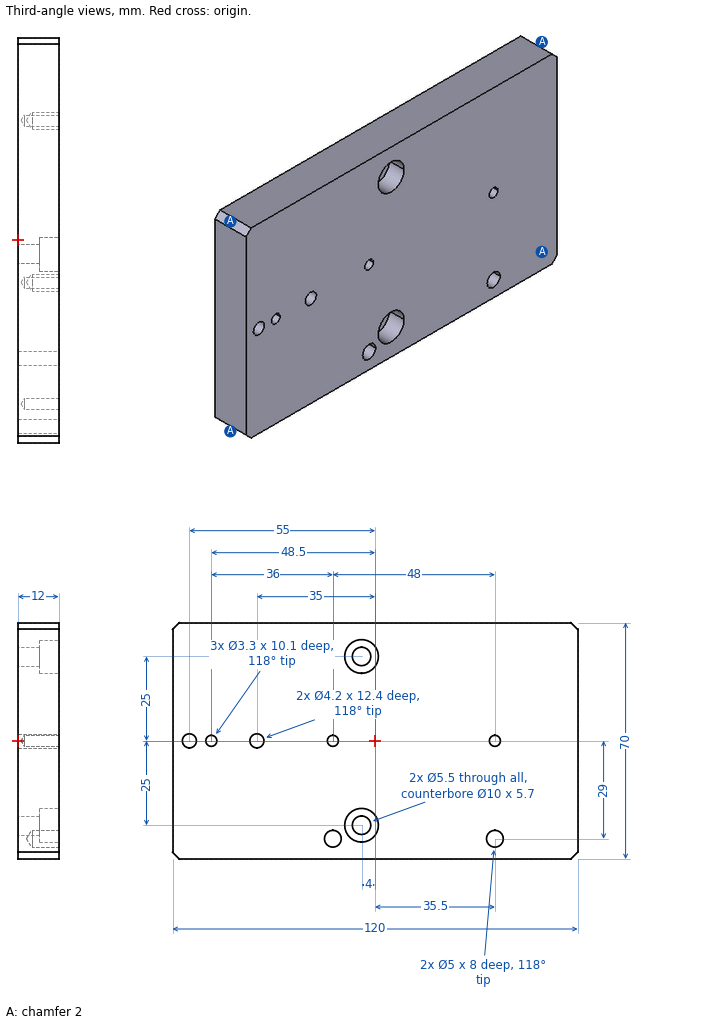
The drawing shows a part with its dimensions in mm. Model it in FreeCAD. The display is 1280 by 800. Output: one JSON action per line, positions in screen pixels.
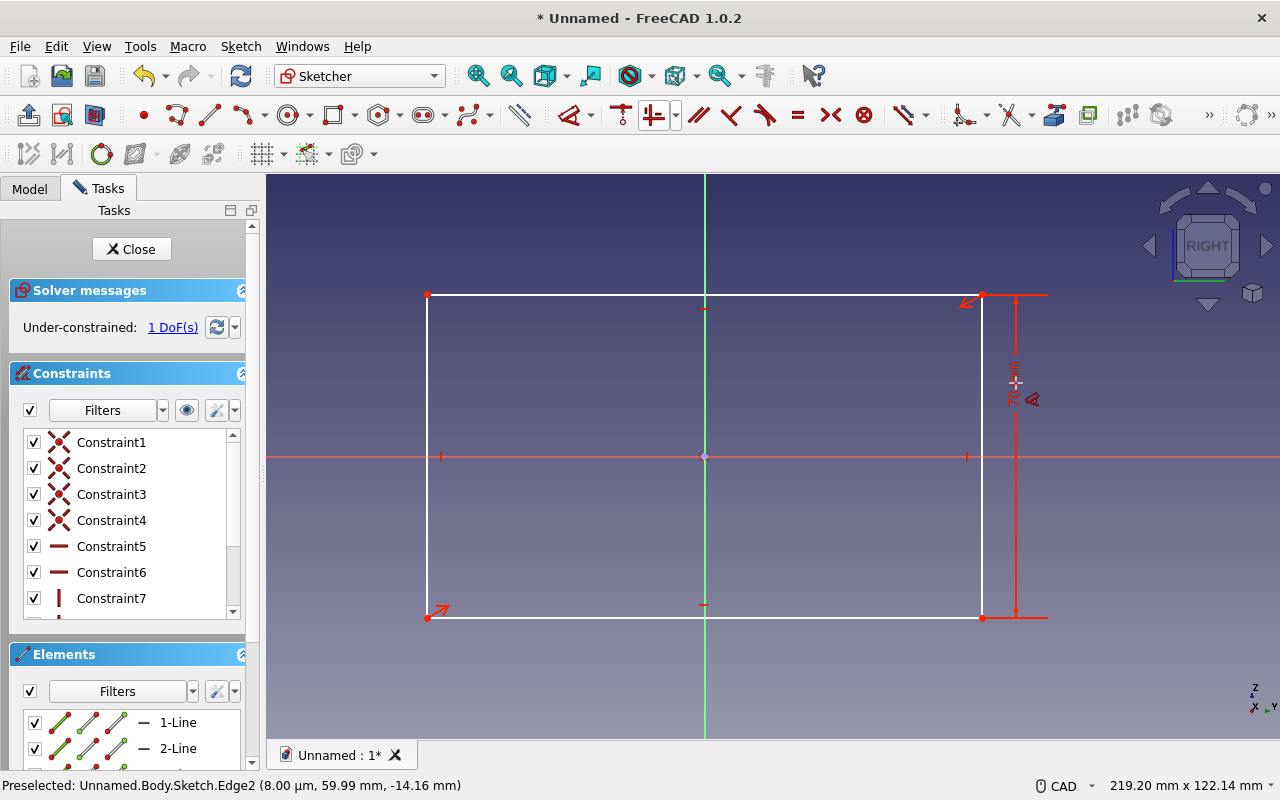
{"action": "left_click", "coordinate": [594, 618]}
{"action": "left_click", "coordinate": [577, 652]}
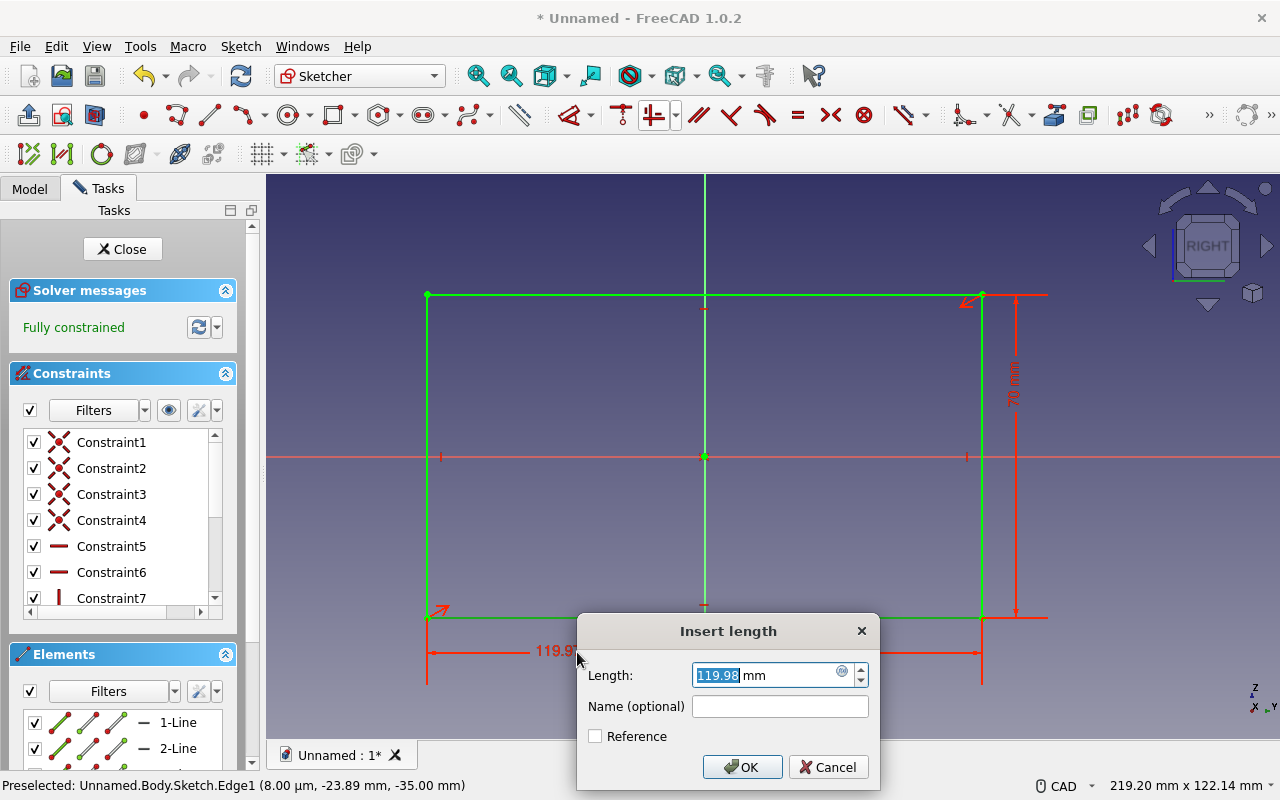
{"action": "type", "text": "120"}
{"action": "key", "text": "Return"}
{"action": "key", "text": "Escape"}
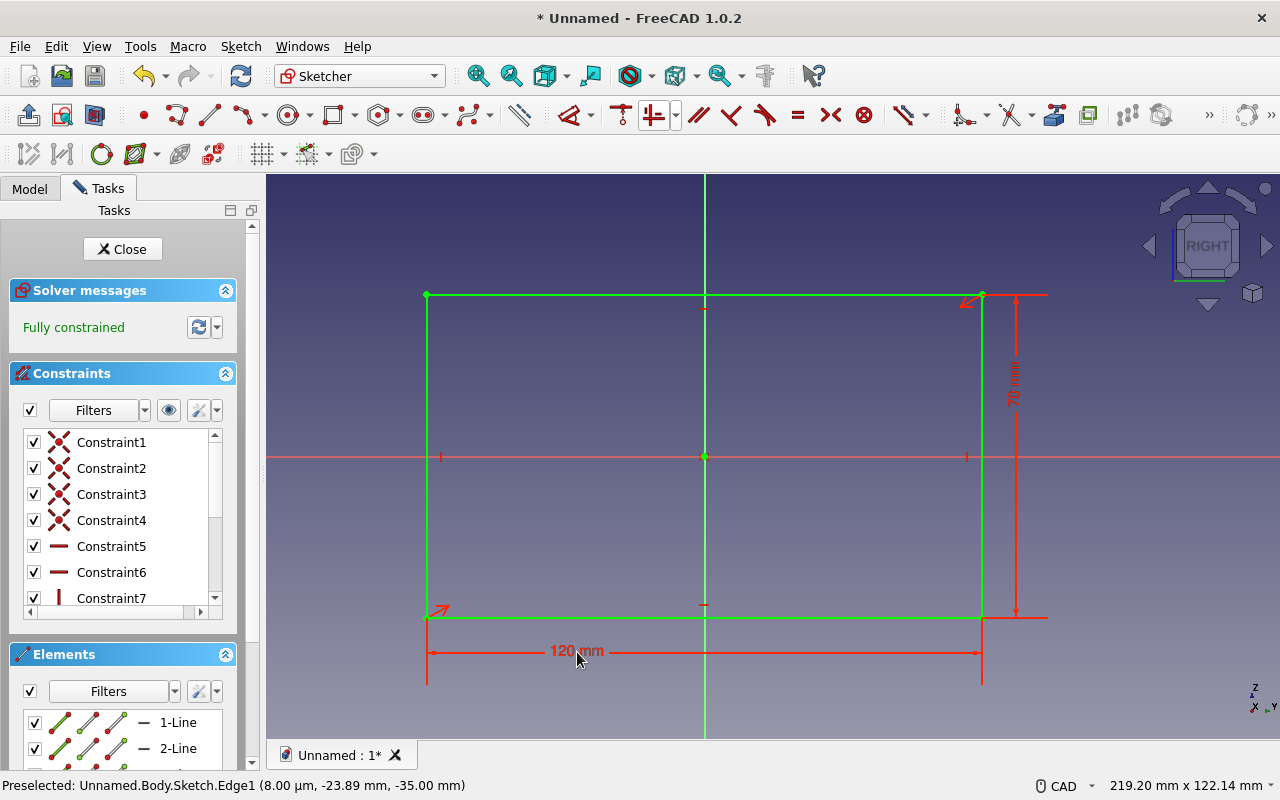
{"action": "left_click", "coordinate": [123, 249]}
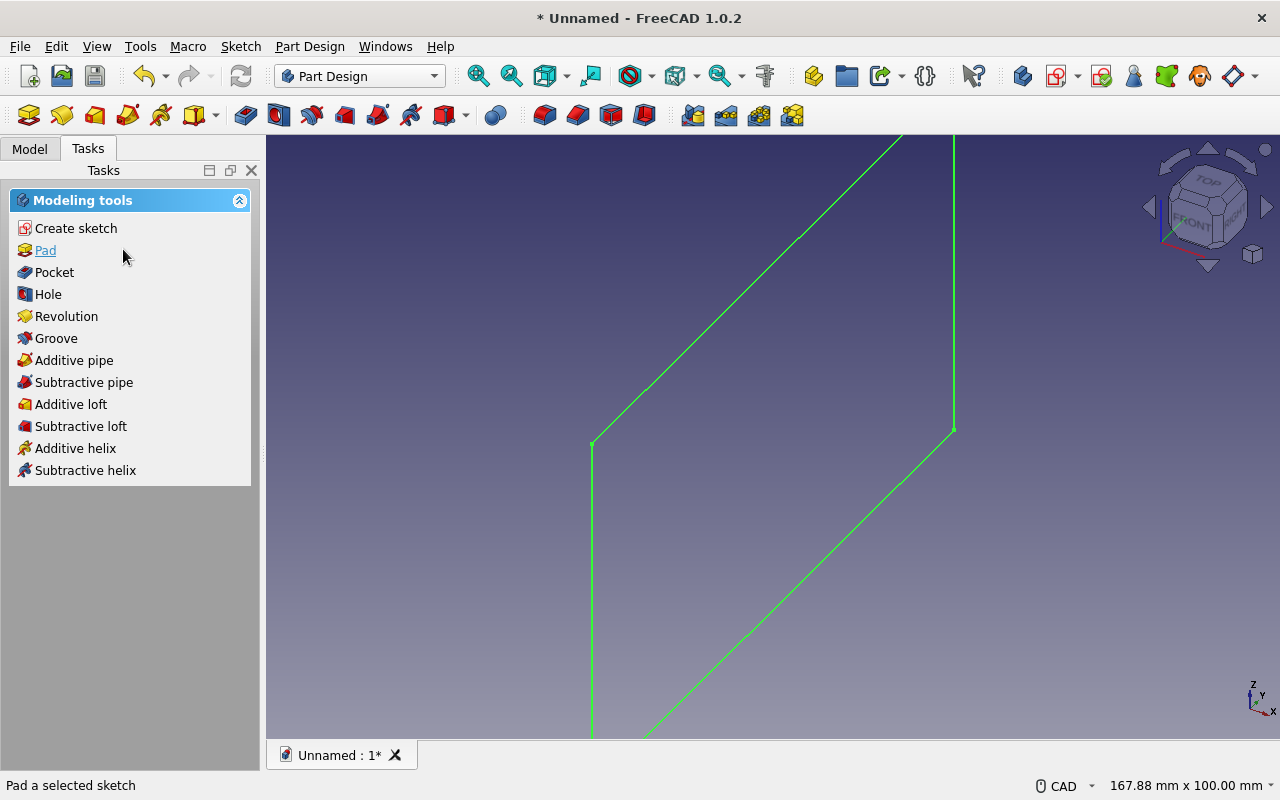
{"action": "left_click", "coordinate": [29, 116]}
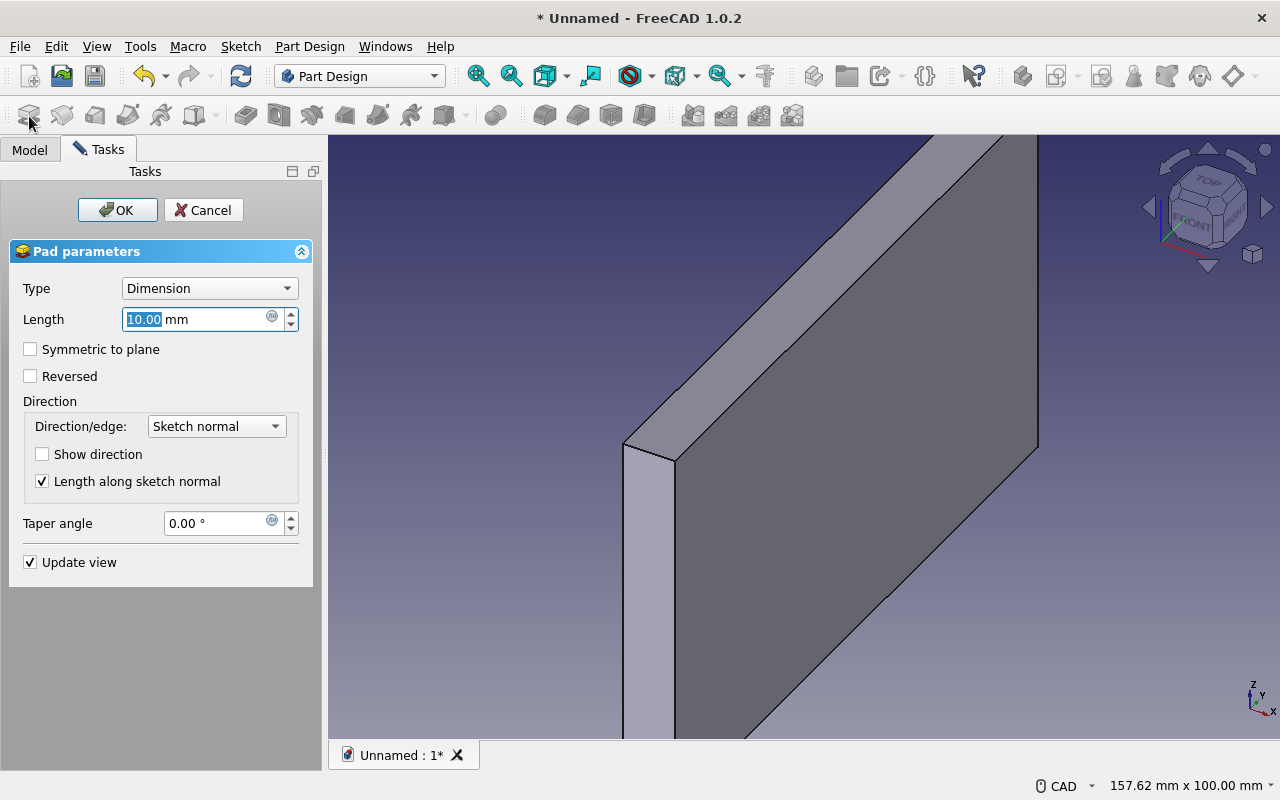
{"action": "type", "text": "12"}
{"action": "key", "text": "Tab"}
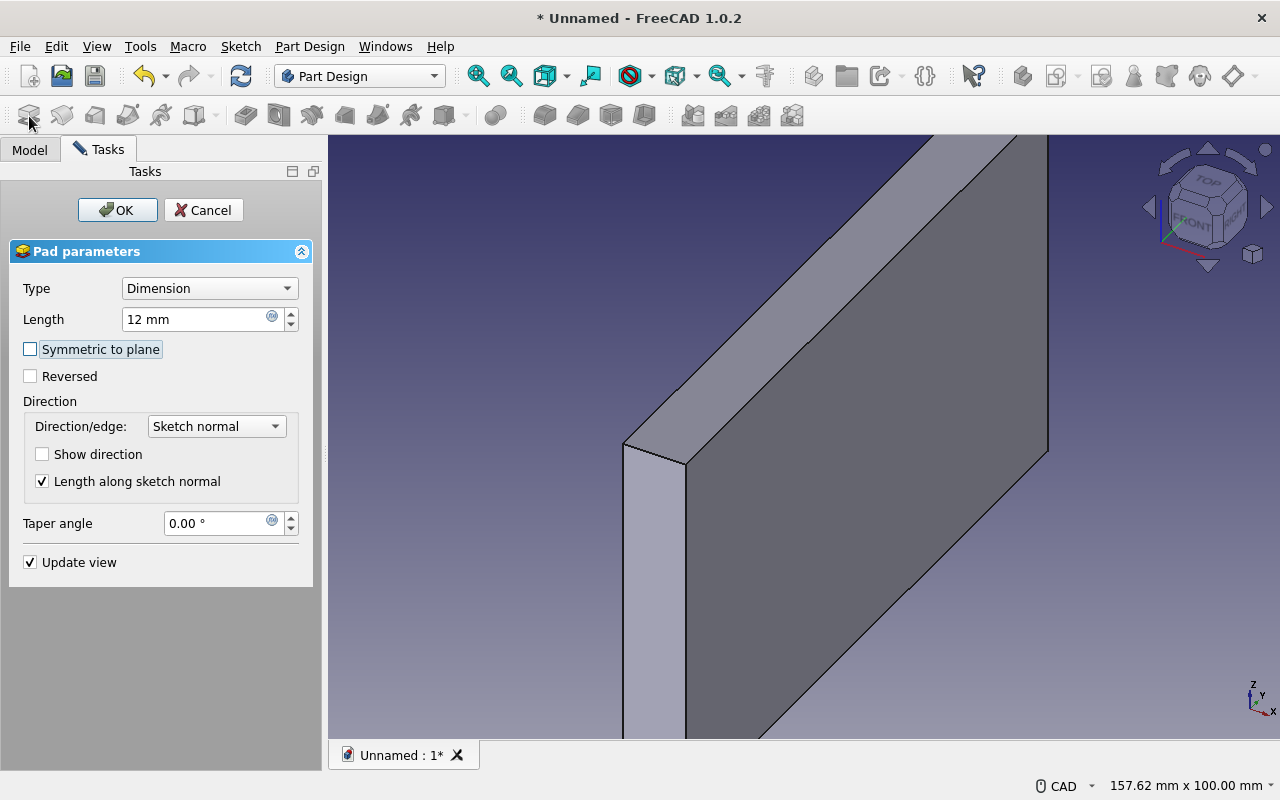
{"action": "left_click", "coordinate": [118, 210]}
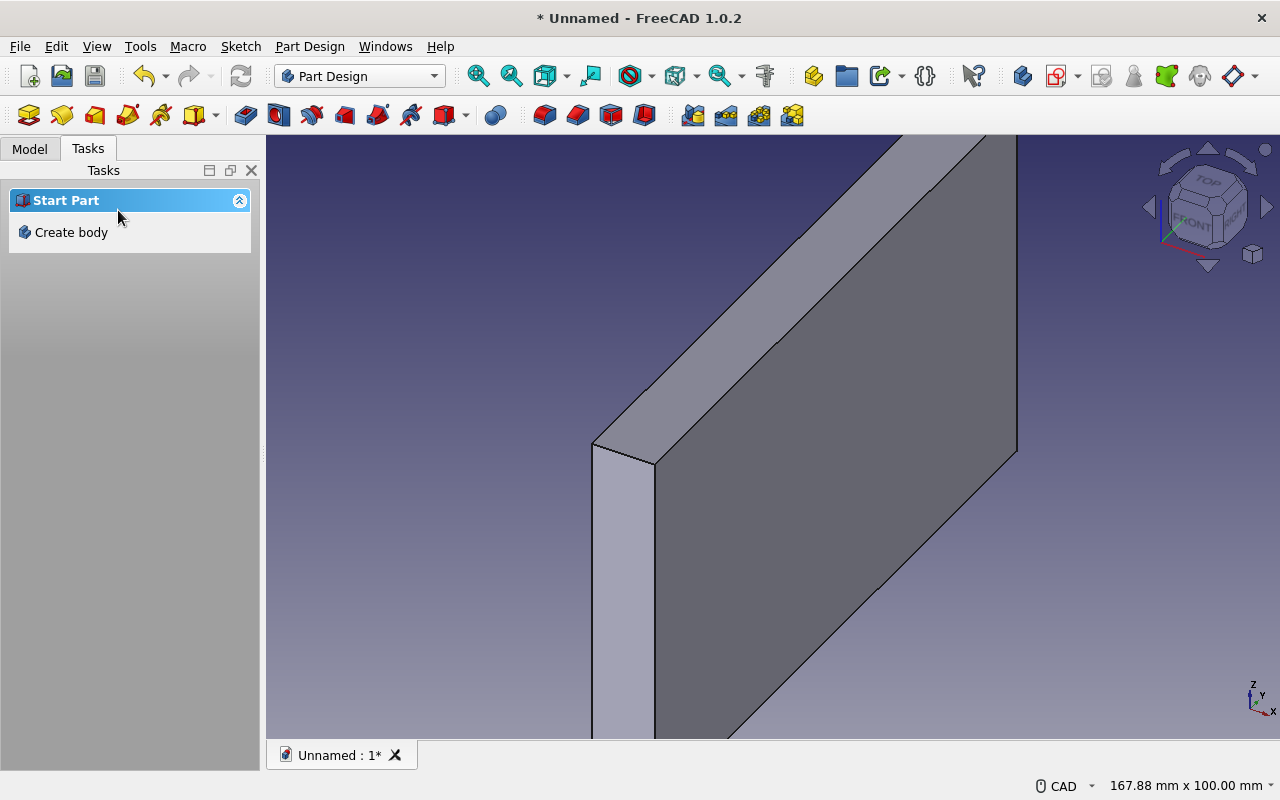
{"action": "left_click", "coordinate": [479, 76]}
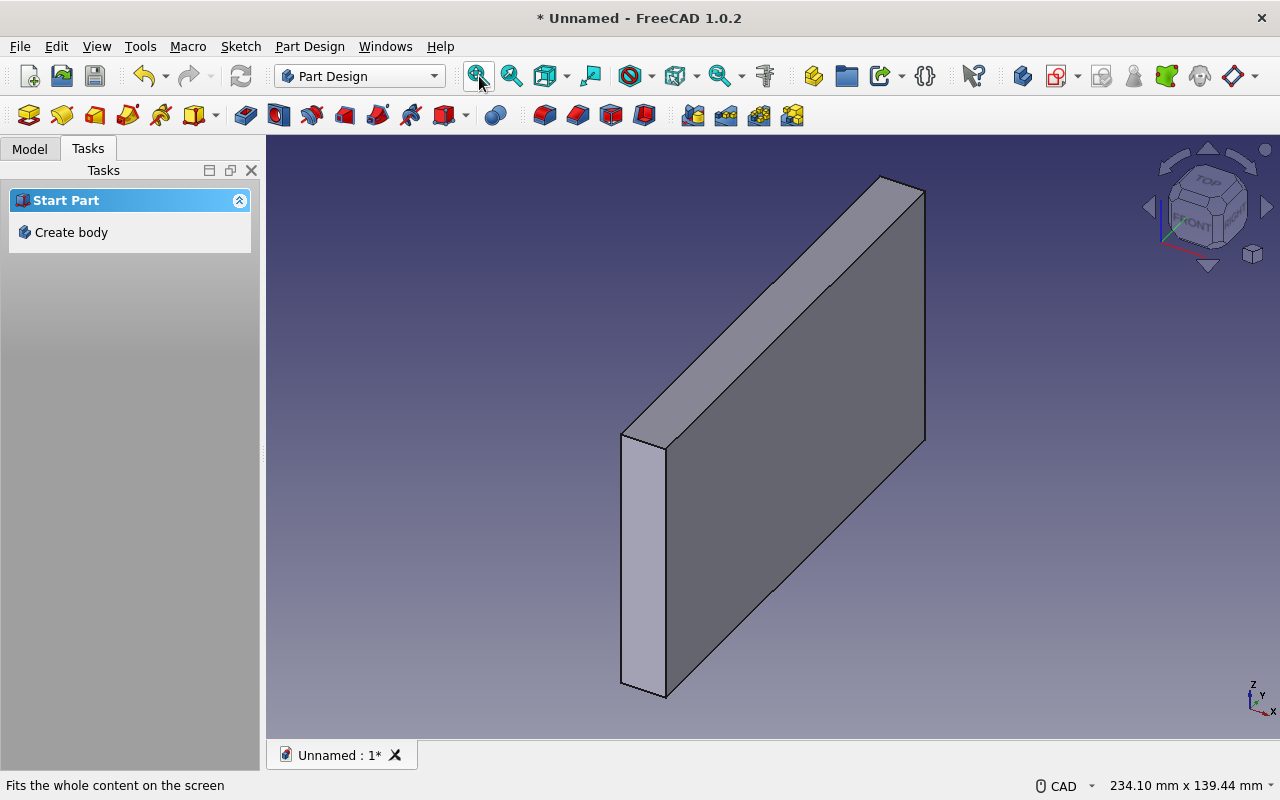
{"action": "key", "text": "6"}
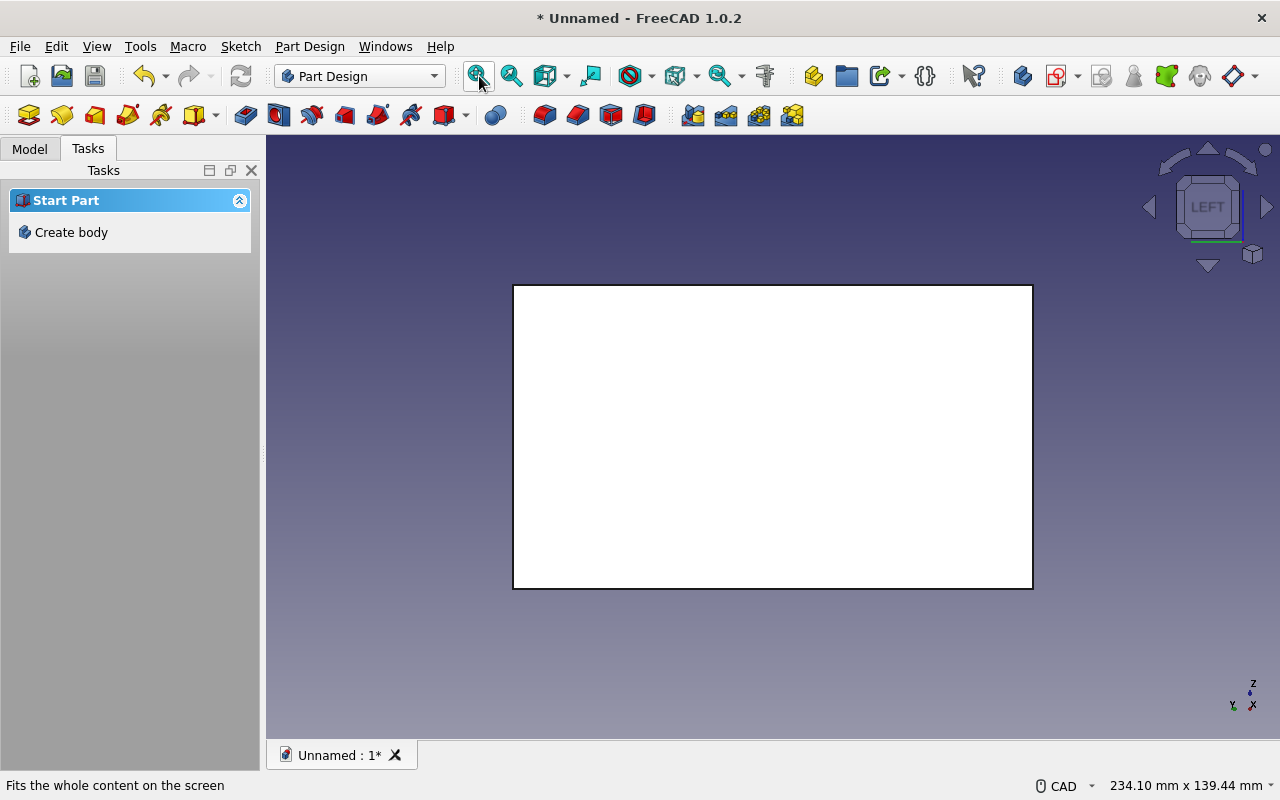
{"action": "left_click", "coordinate": [699, 436]}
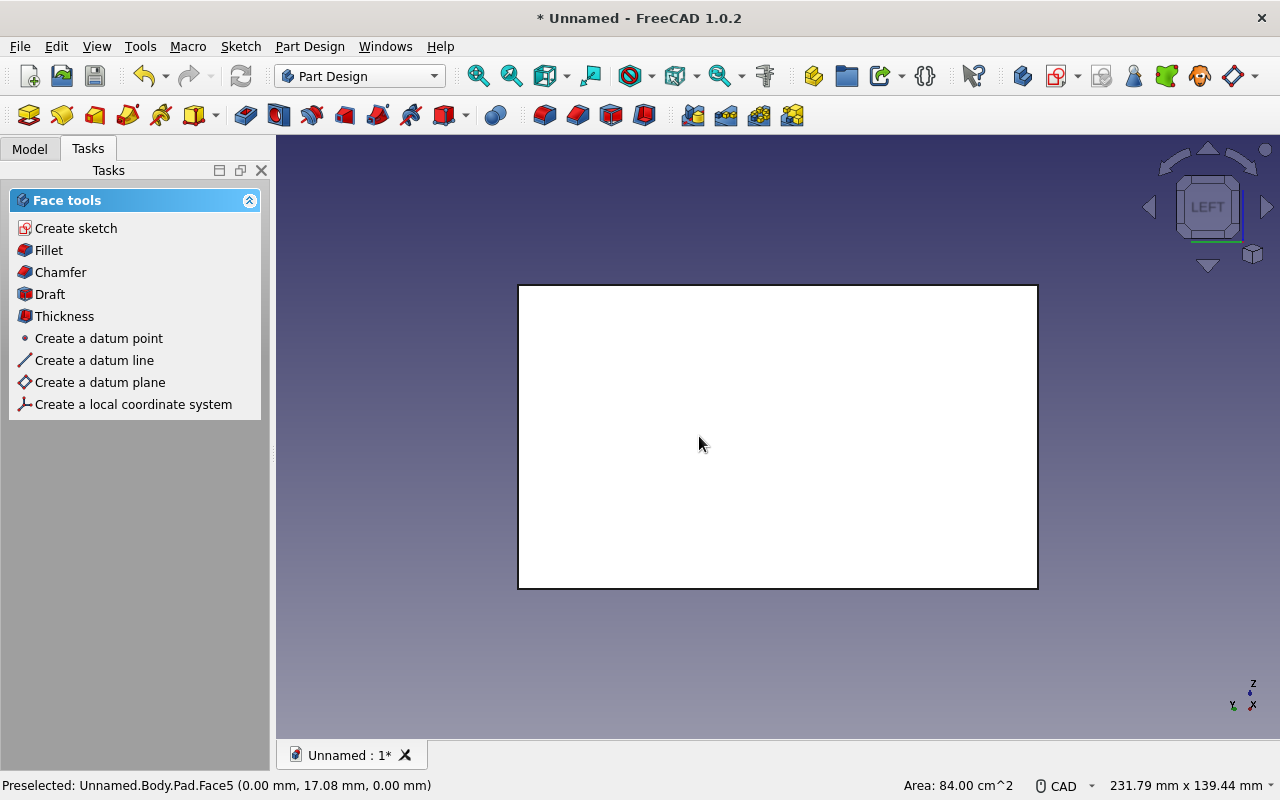
{"action": "left_click", "coordinate": [1056, 76]}